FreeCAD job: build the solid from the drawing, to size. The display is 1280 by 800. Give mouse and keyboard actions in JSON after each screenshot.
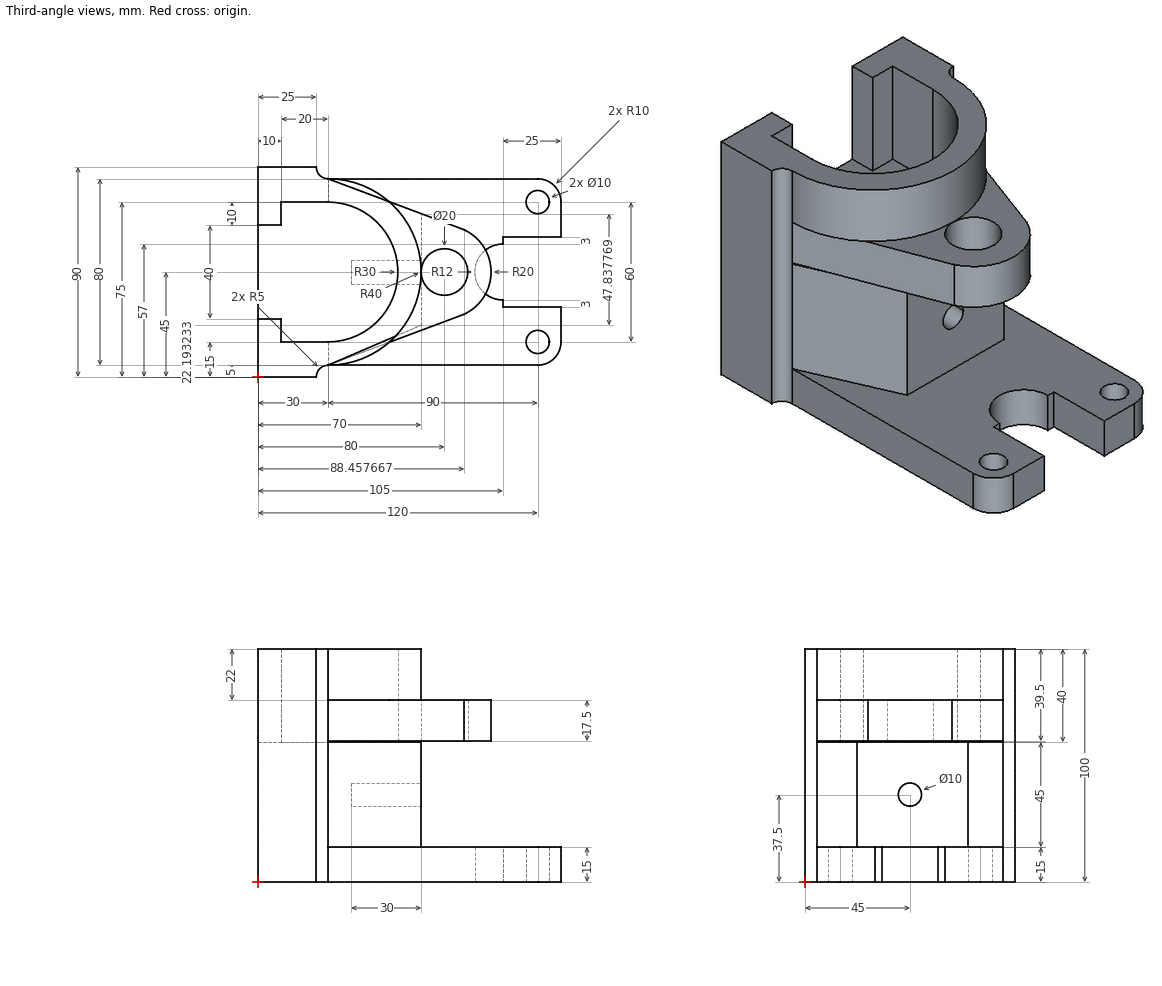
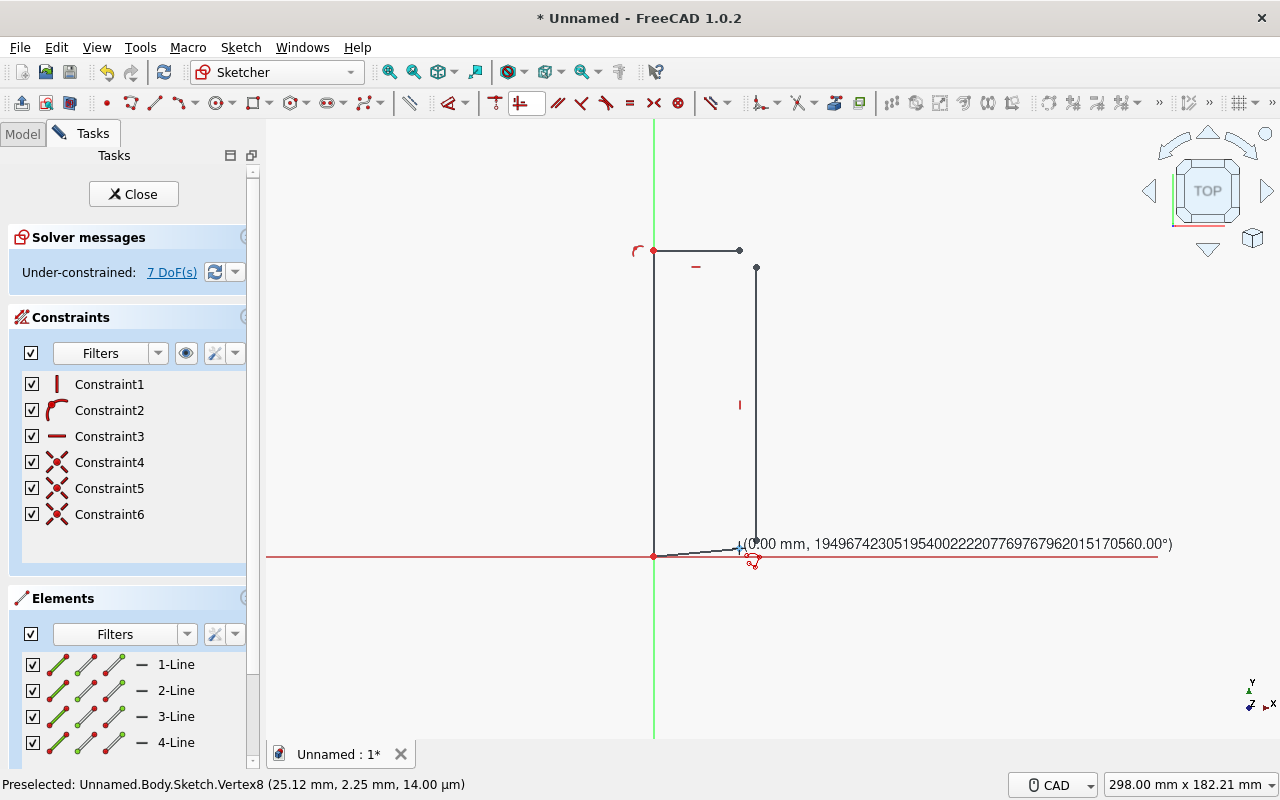
{"action": "left_click", "coordinate": [180, 104]}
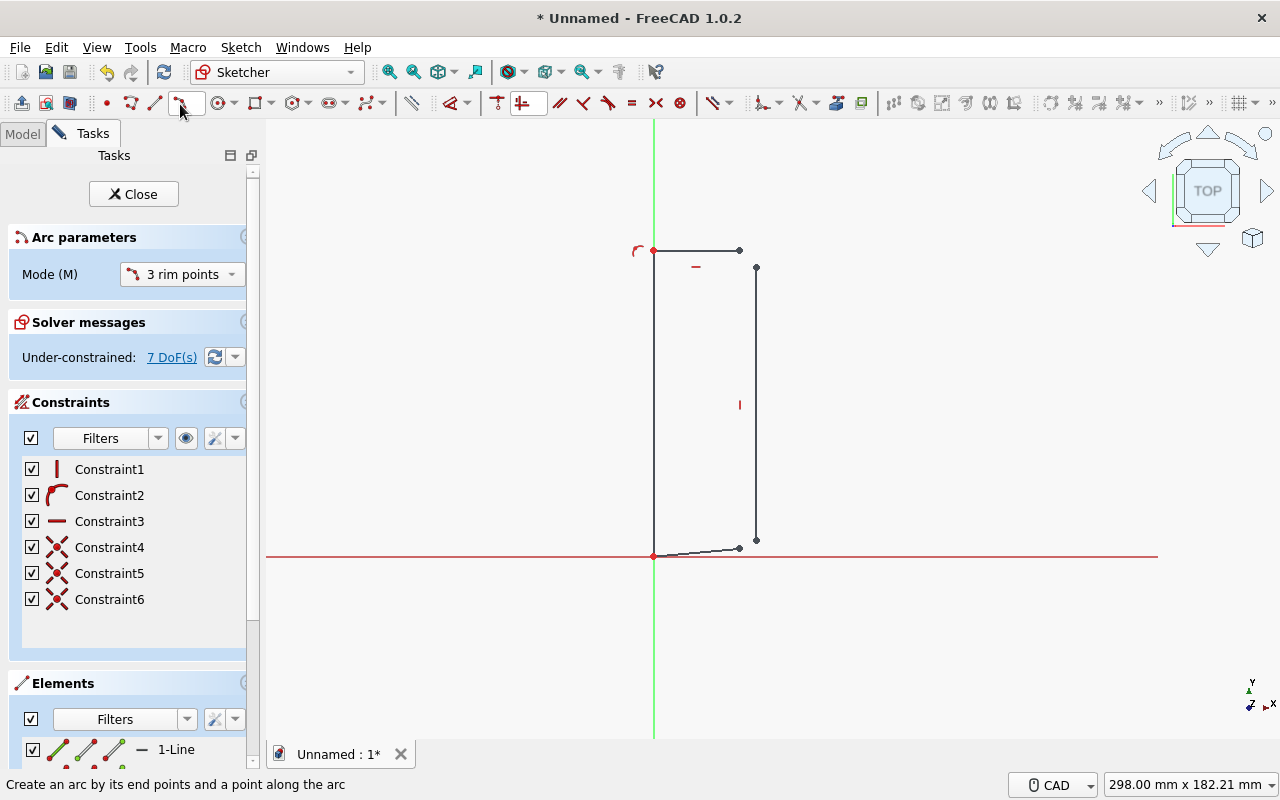
{"action": "left_click", "coordinate": [756, 268]}
{"action": "left_click", "coordinate": [739, 251]}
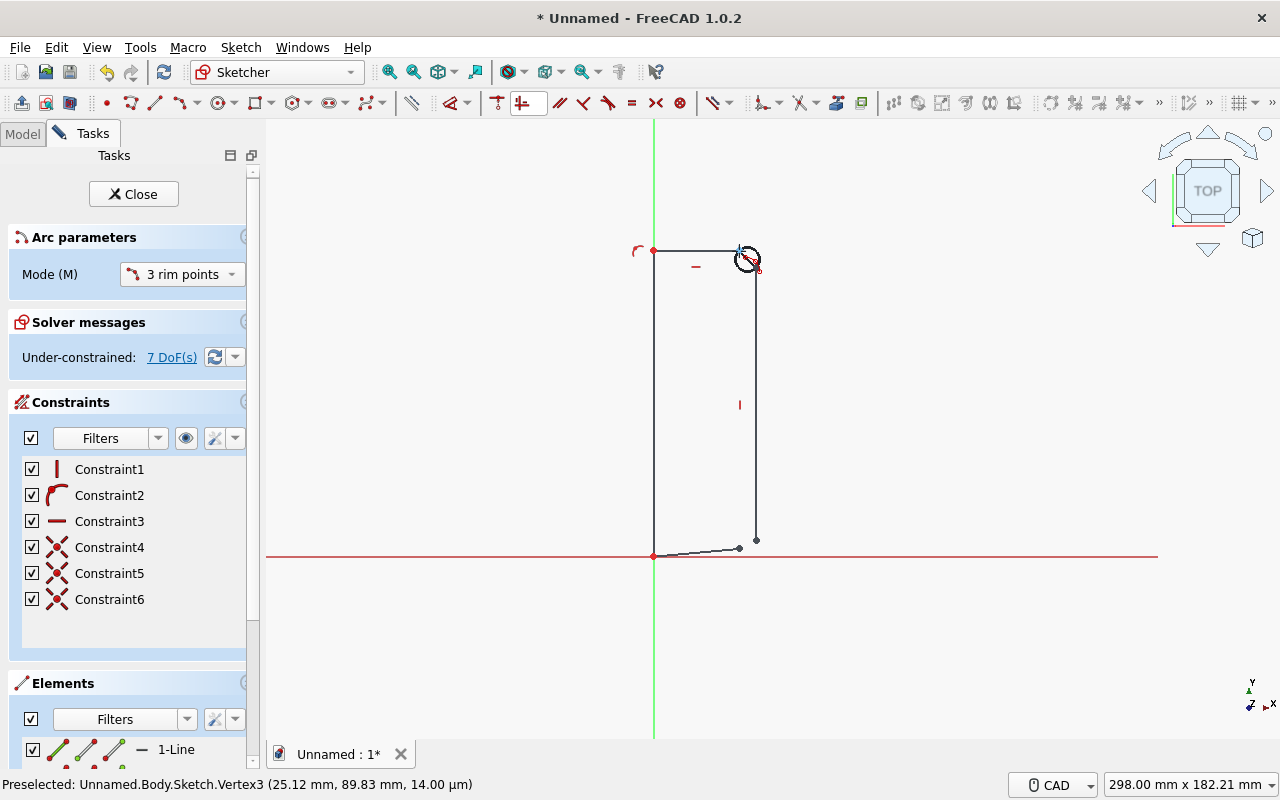
{"action": "scroll", "coordinate": [744, 262], "scroll_direction": "up", "scroll_amount": 6}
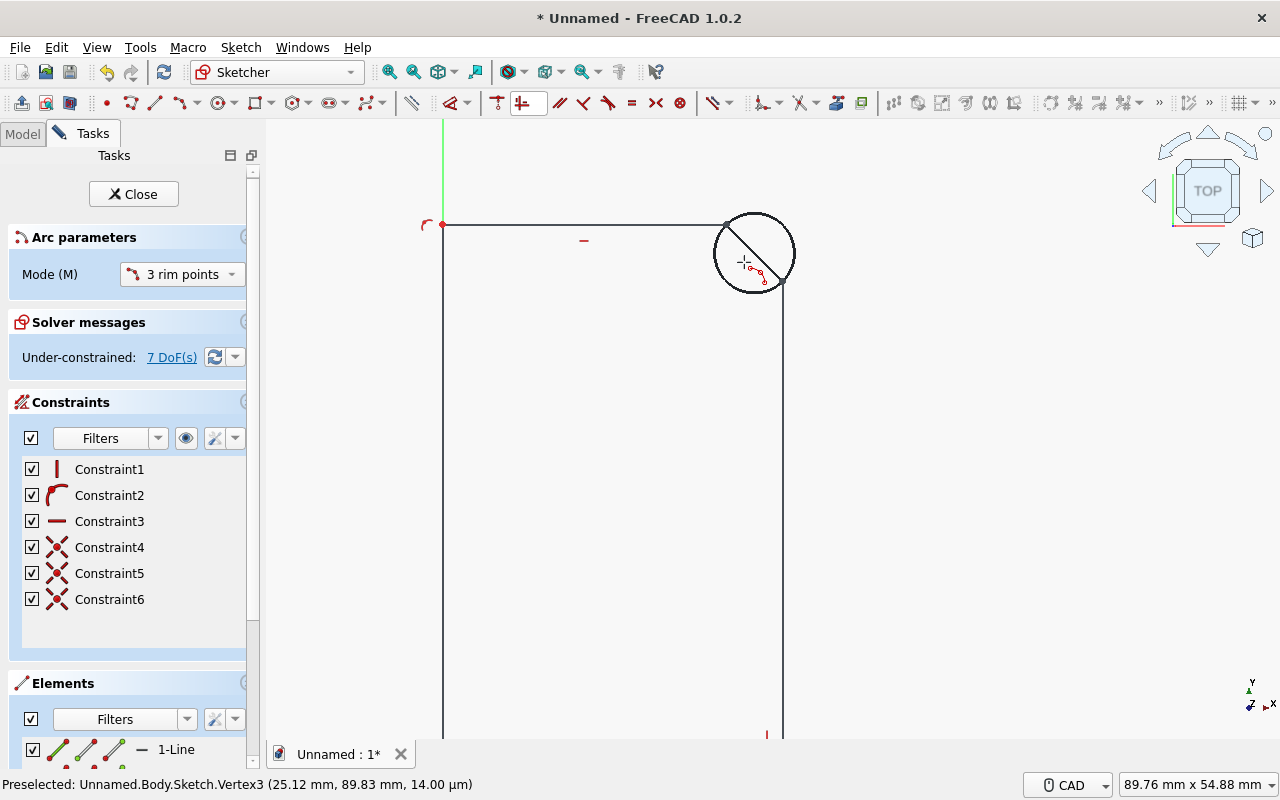
{"action": "left_click", "coordinate": [742, 263]}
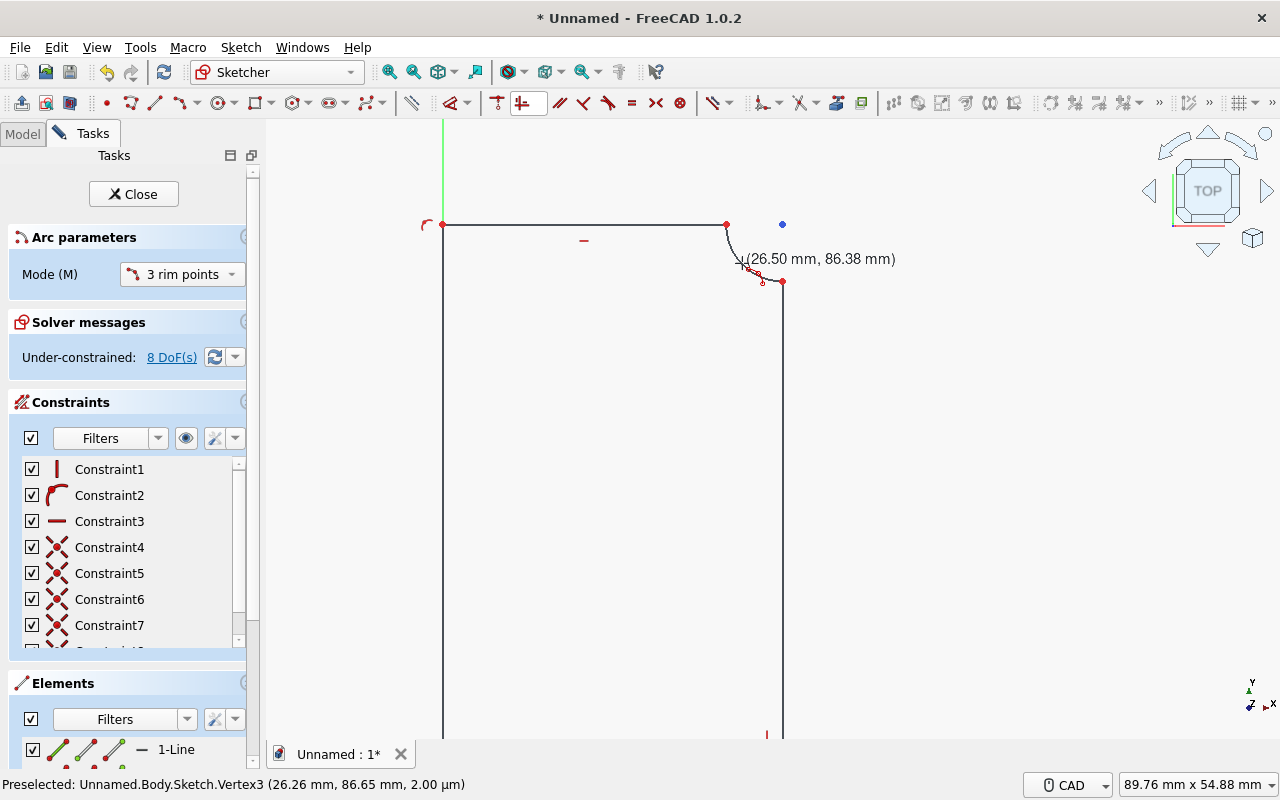
{"action": "scroll", "coordinate": [758, 253], "scroll_direction": "down", "scroll_amount": 5}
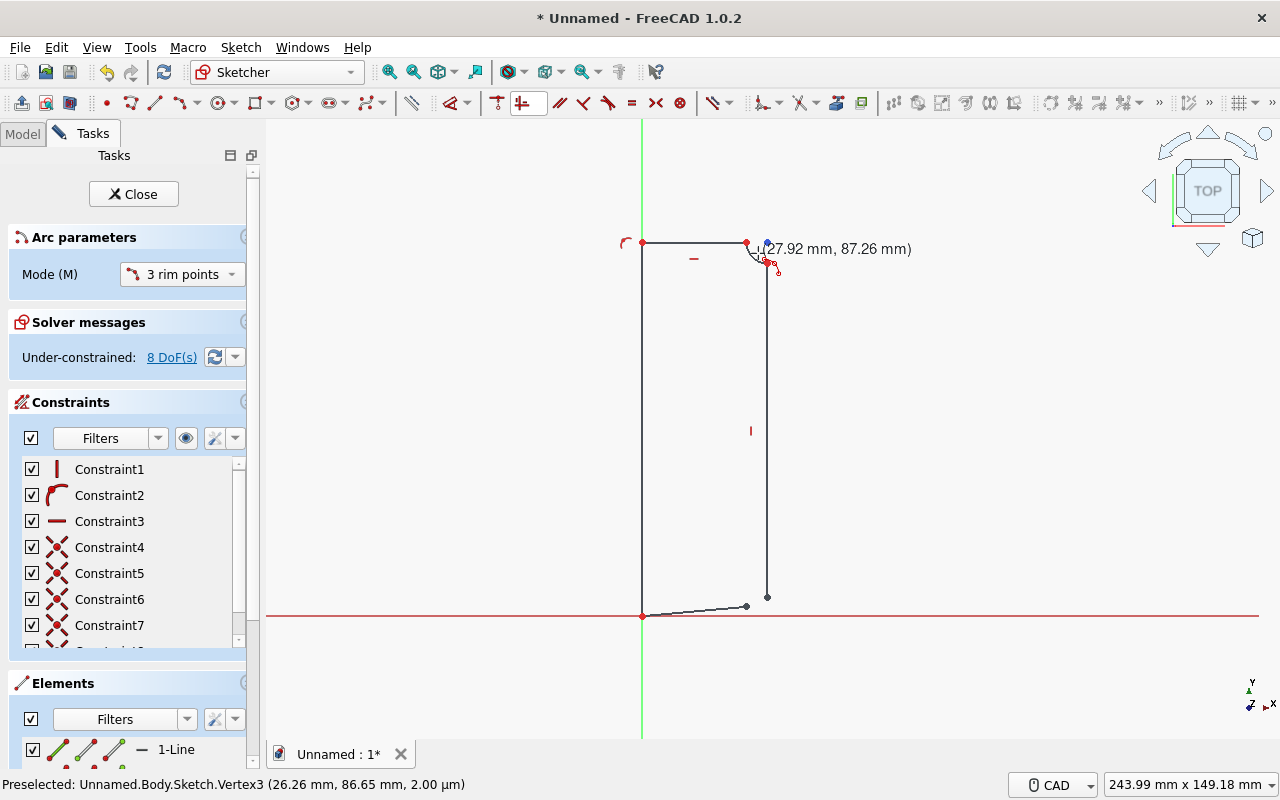
{"action": "left_click", "coordinate": [747, 607]}
{"action": "left_click", "coordinate": [767, 597]}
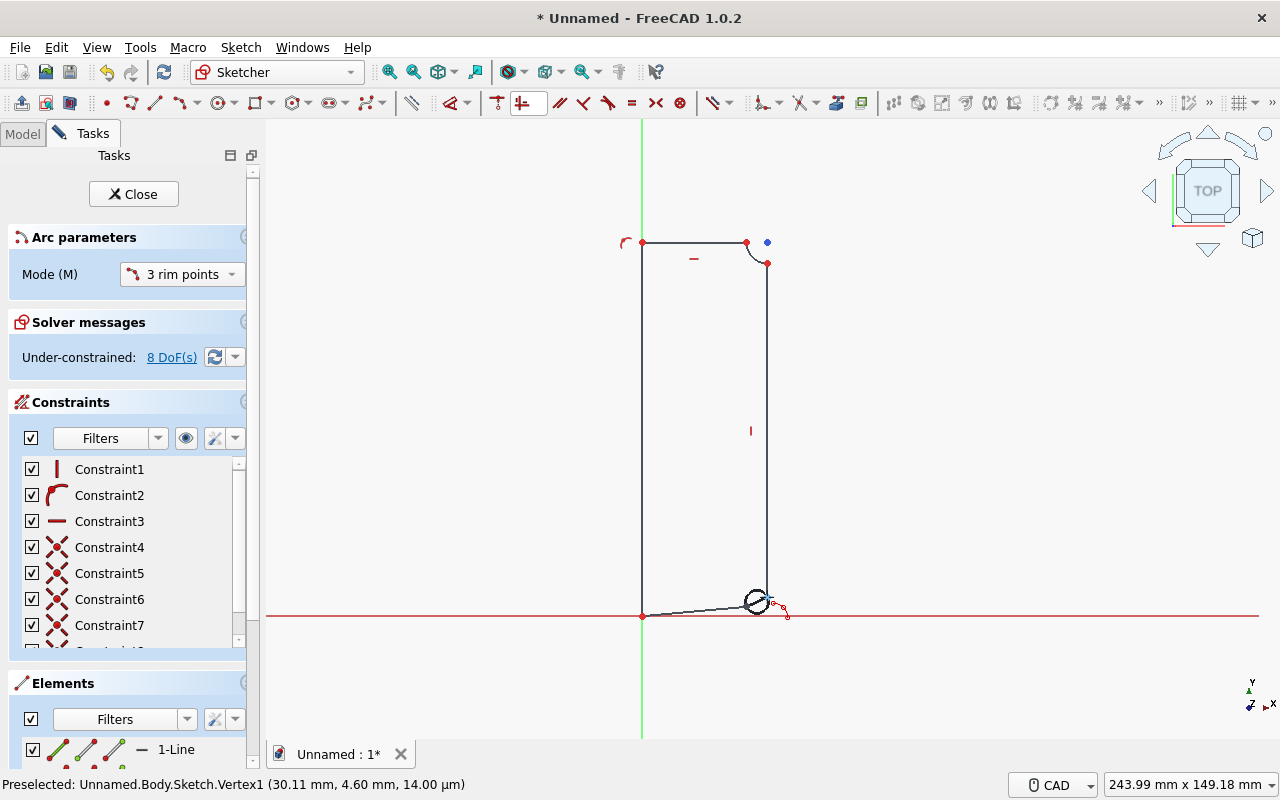
{"action": "scroll", "coordinate": [752, 601], "scroll_direction": "up", "scroll_amount": 5}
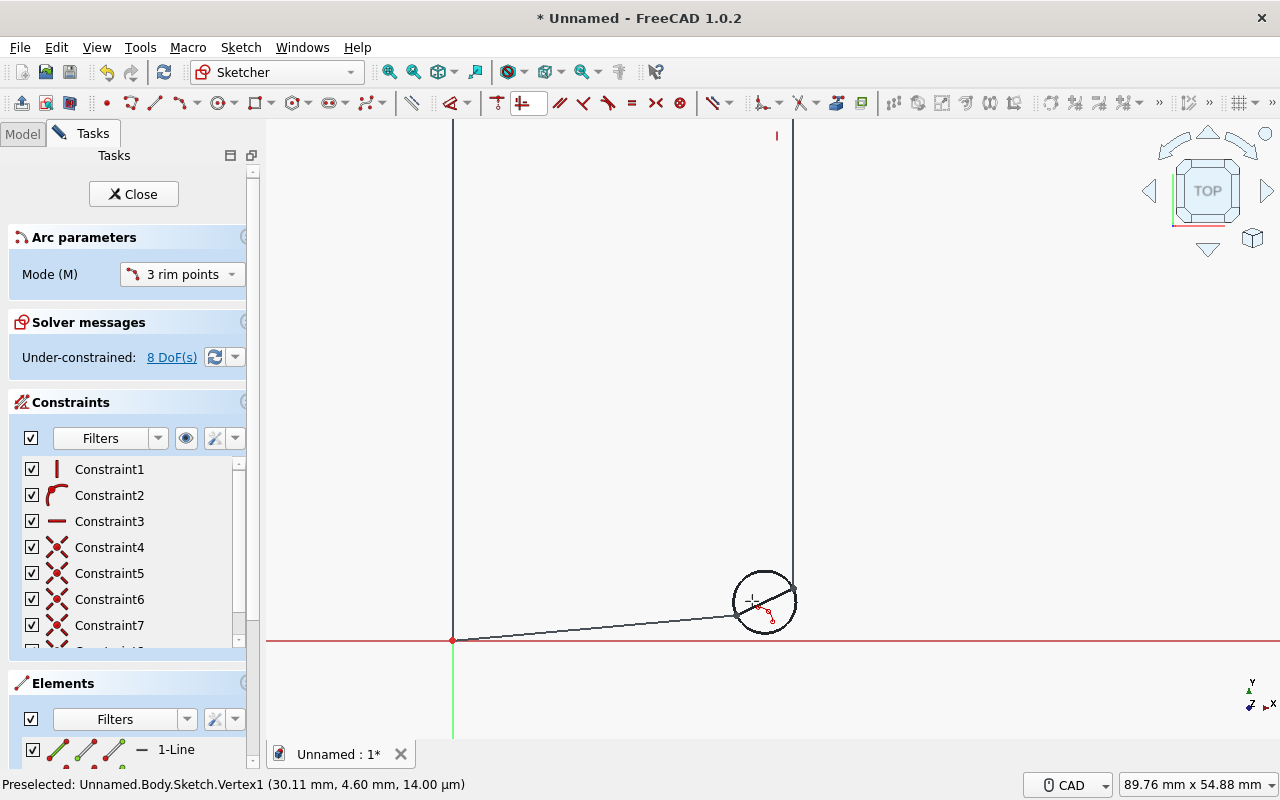
{"action": "left_click", "coordinate": [752, 601]}
{"action": "key", "text": "Escape"}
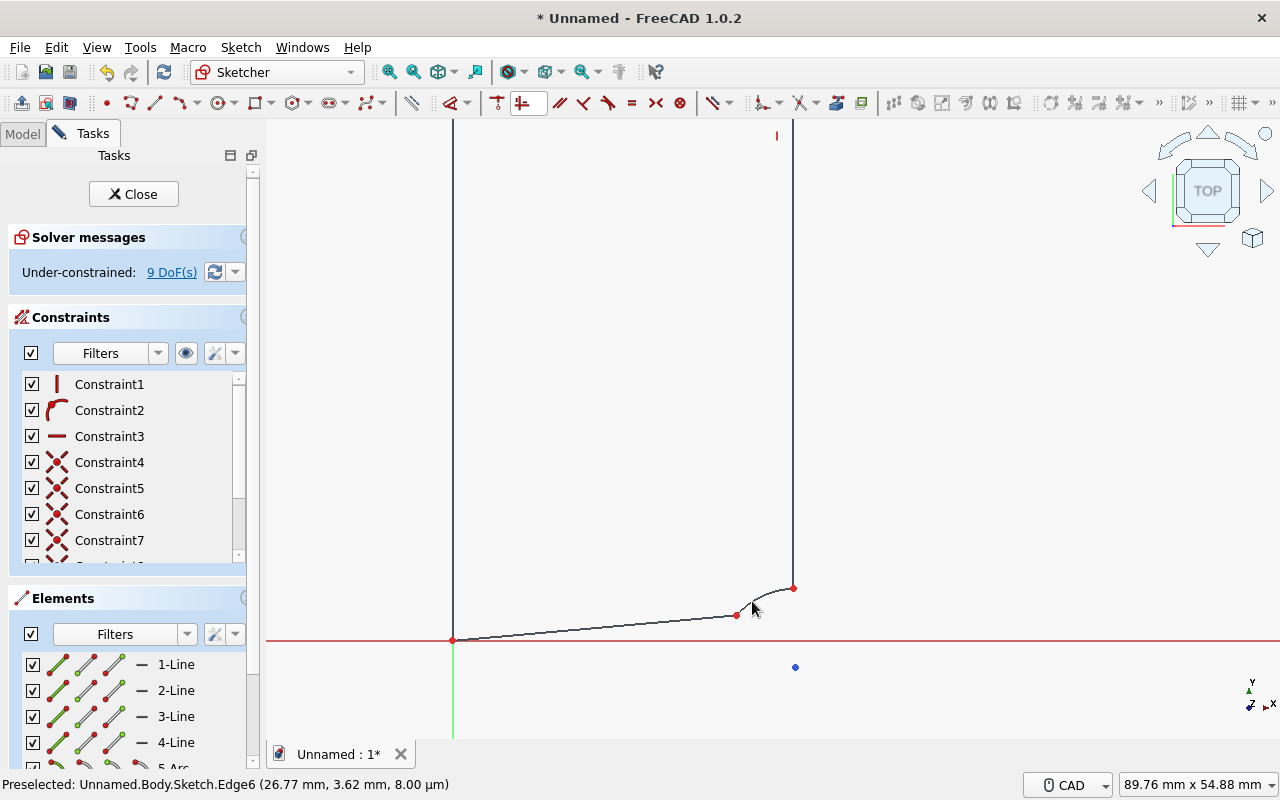
{"action": "left_click", "coordinate": [652, 623]}